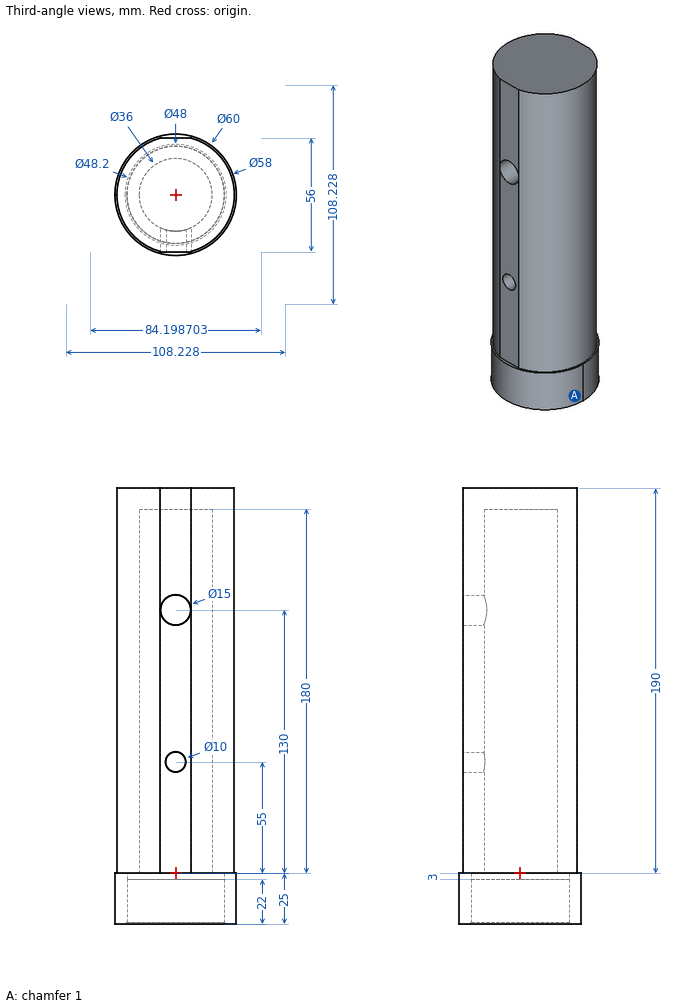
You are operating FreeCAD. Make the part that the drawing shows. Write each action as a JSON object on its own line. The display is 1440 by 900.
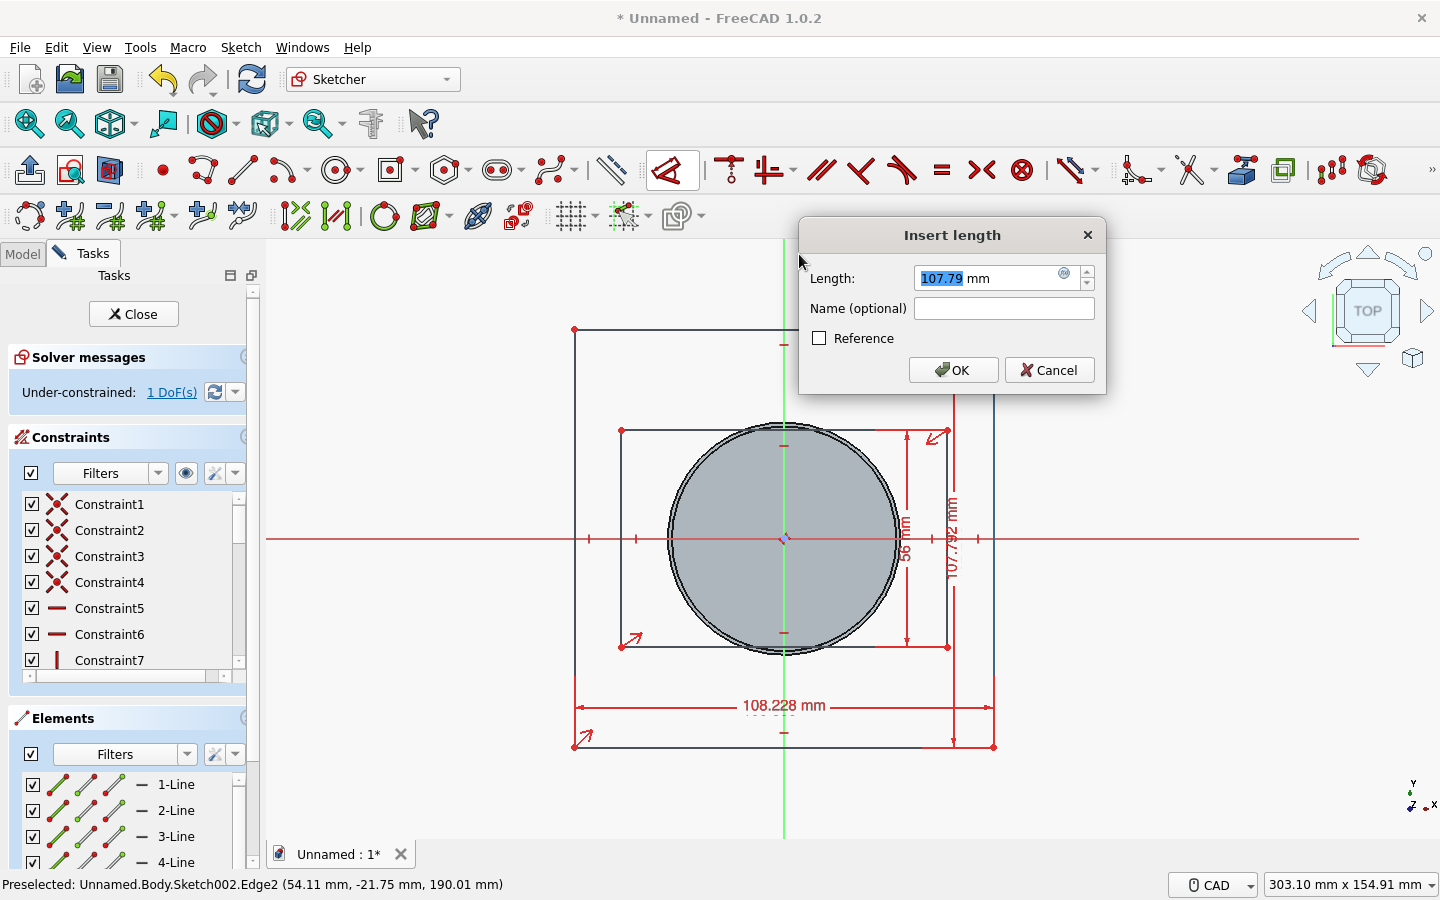
{"action": "type", "text": "108.228"}
{"action": "key", "text": "Return"}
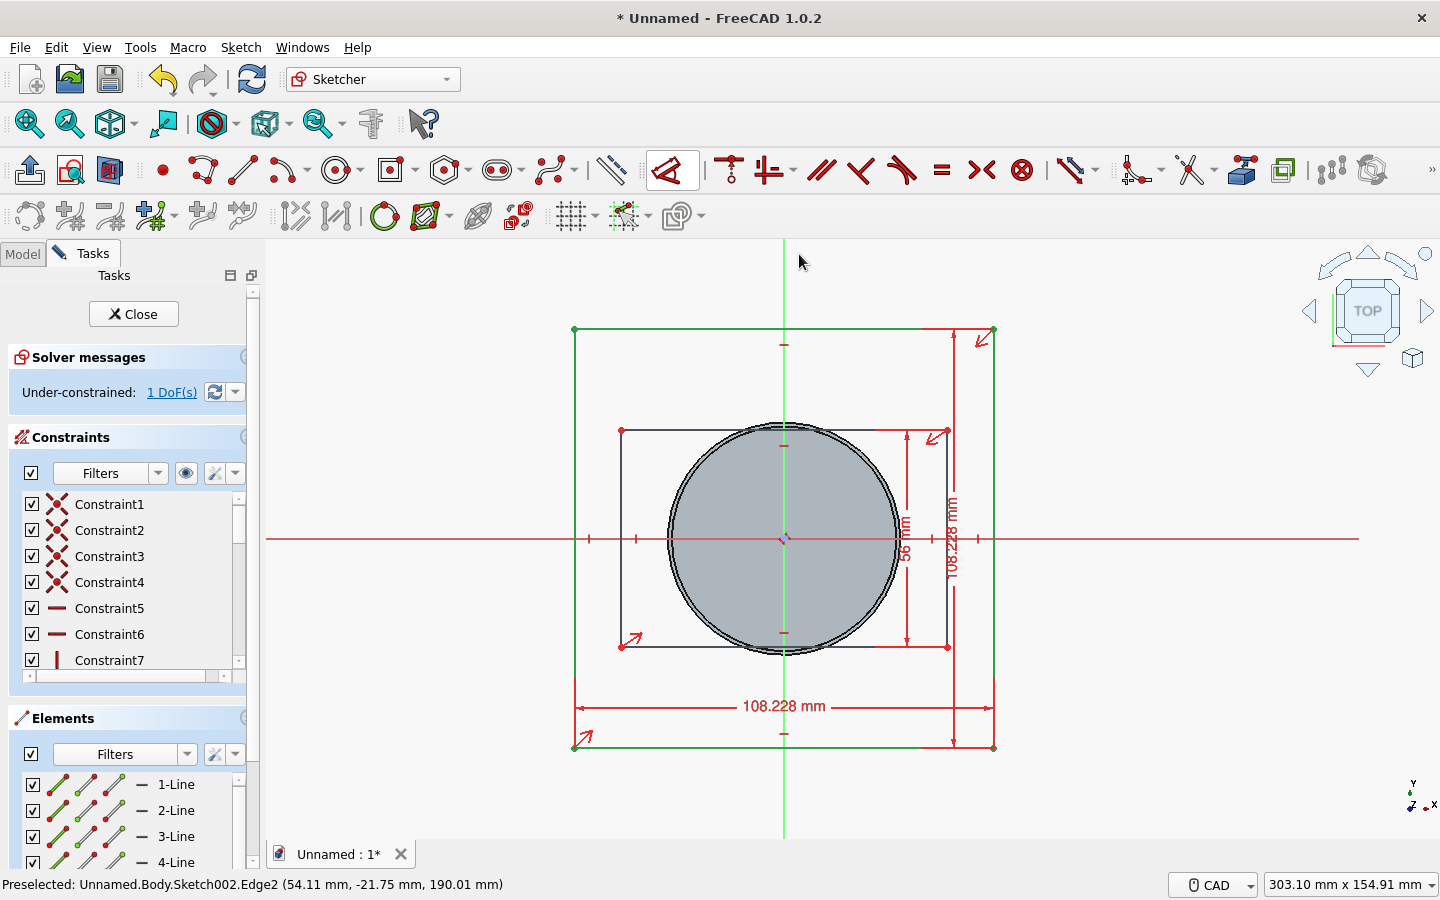
{"action": "left_click", "coordinate": [719, 647]}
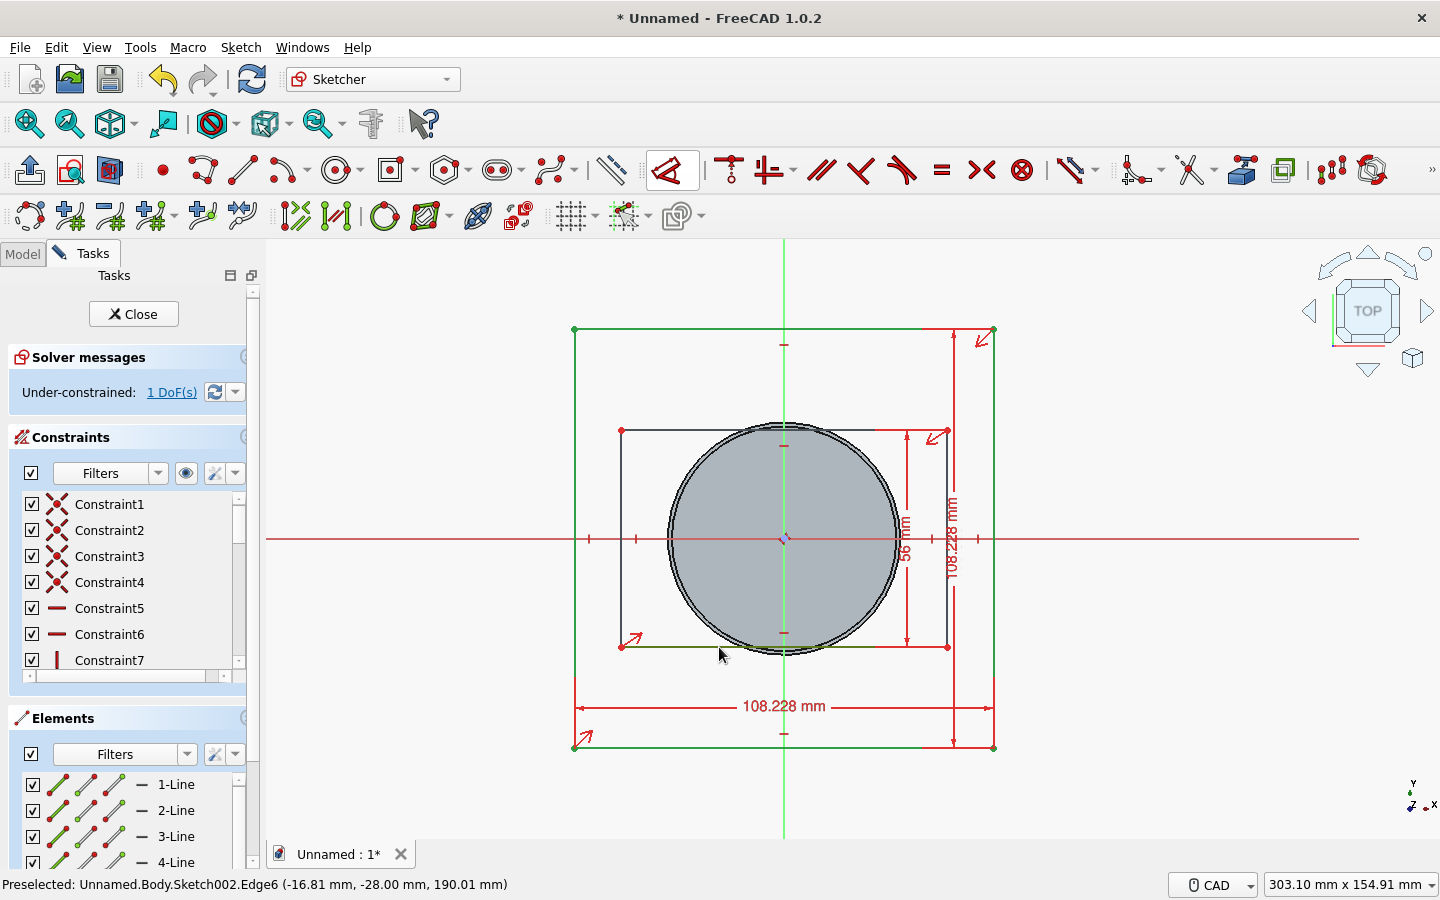
{"action": "key", "text": "l"}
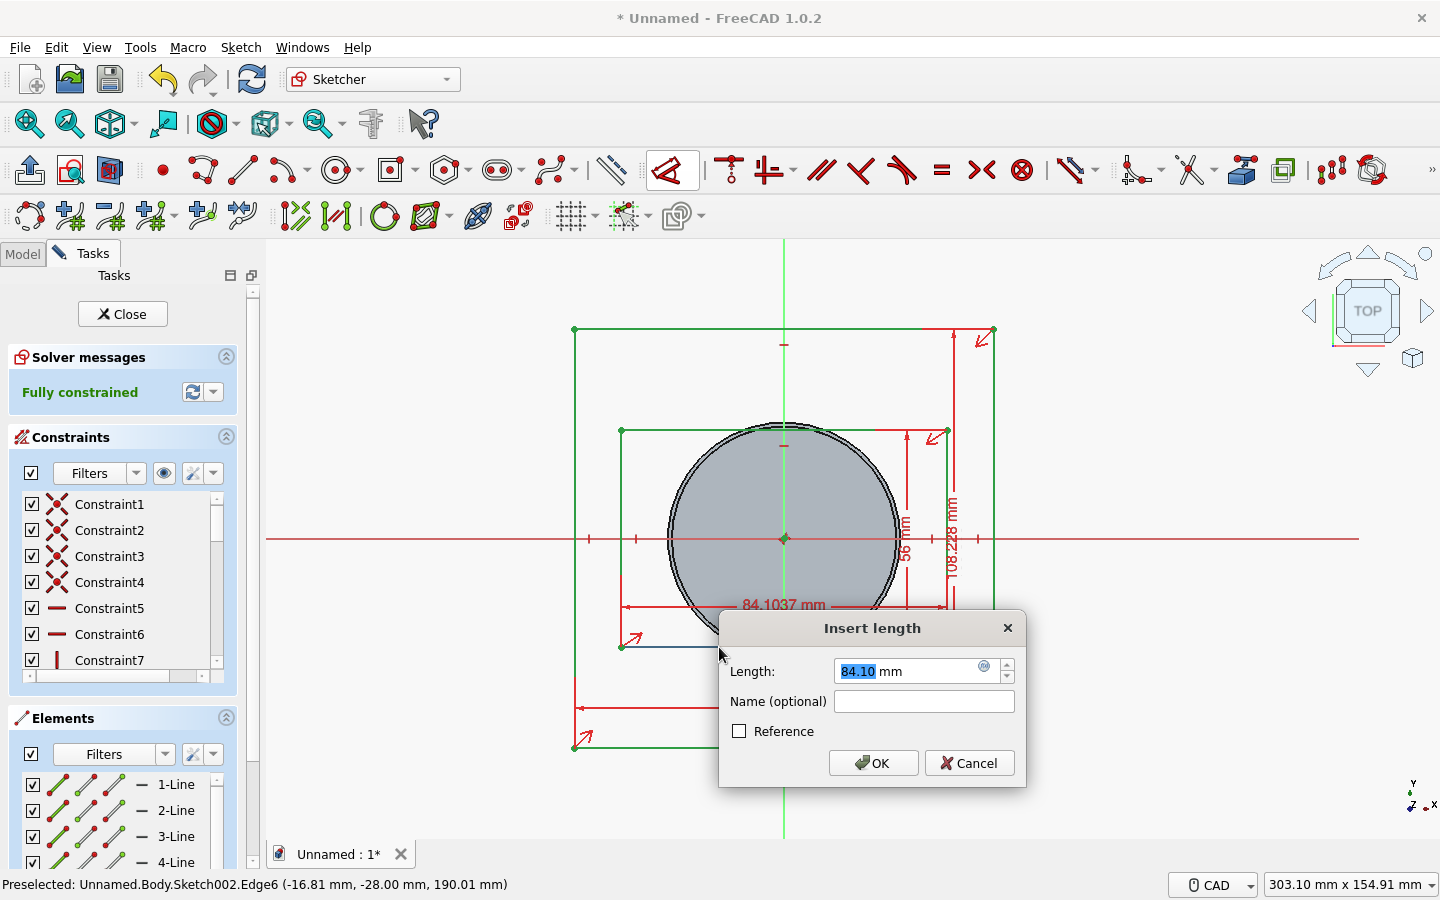
{"action": "type", "text": "84.198703"}
{"action": "key", "text": "Return"}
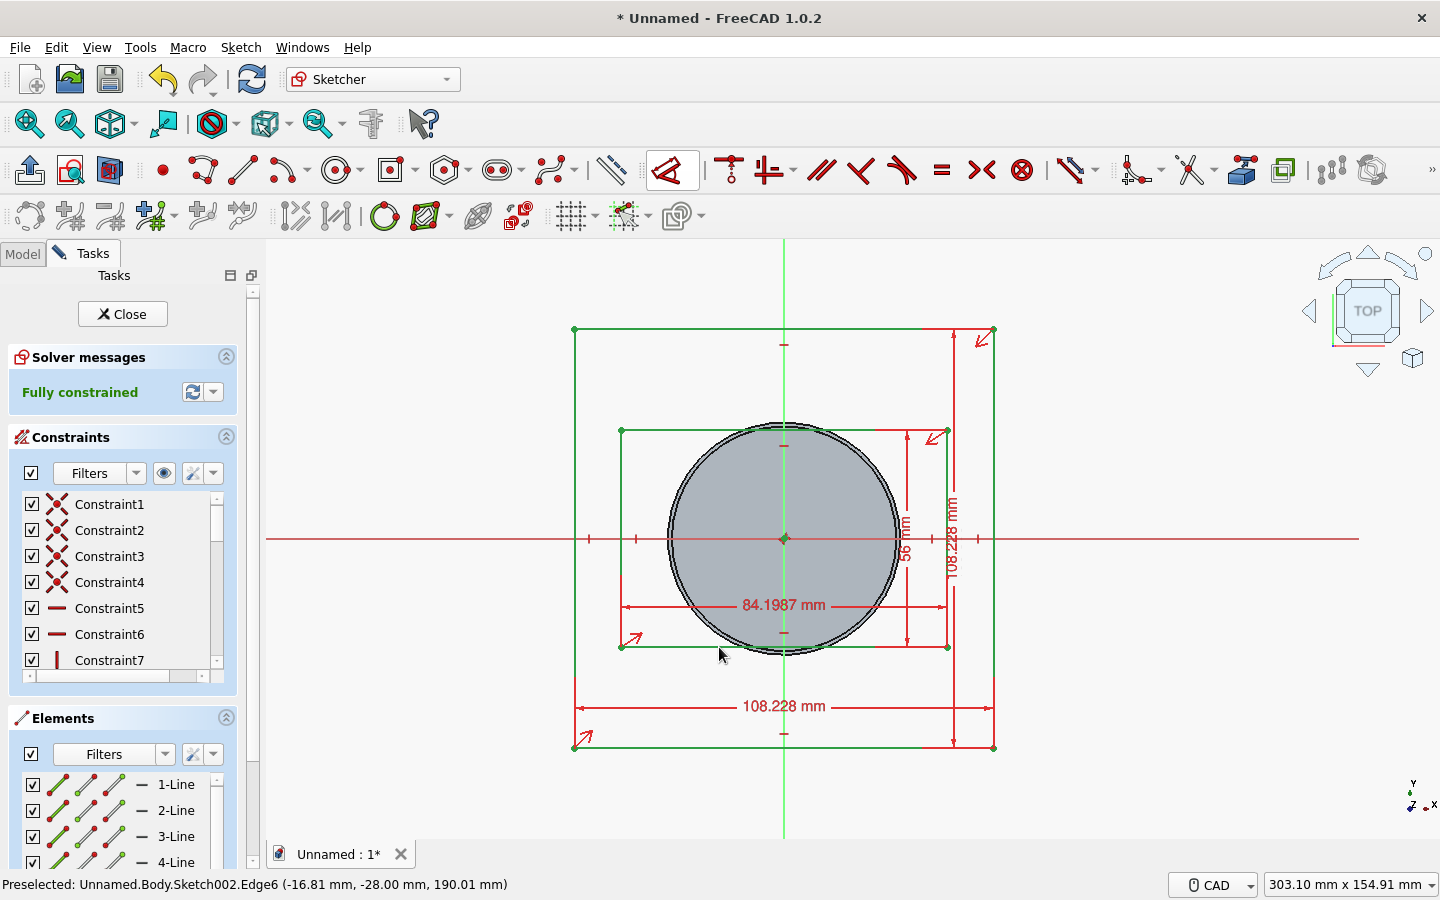
{"action": "left_click", "coordinate": [123, 314]}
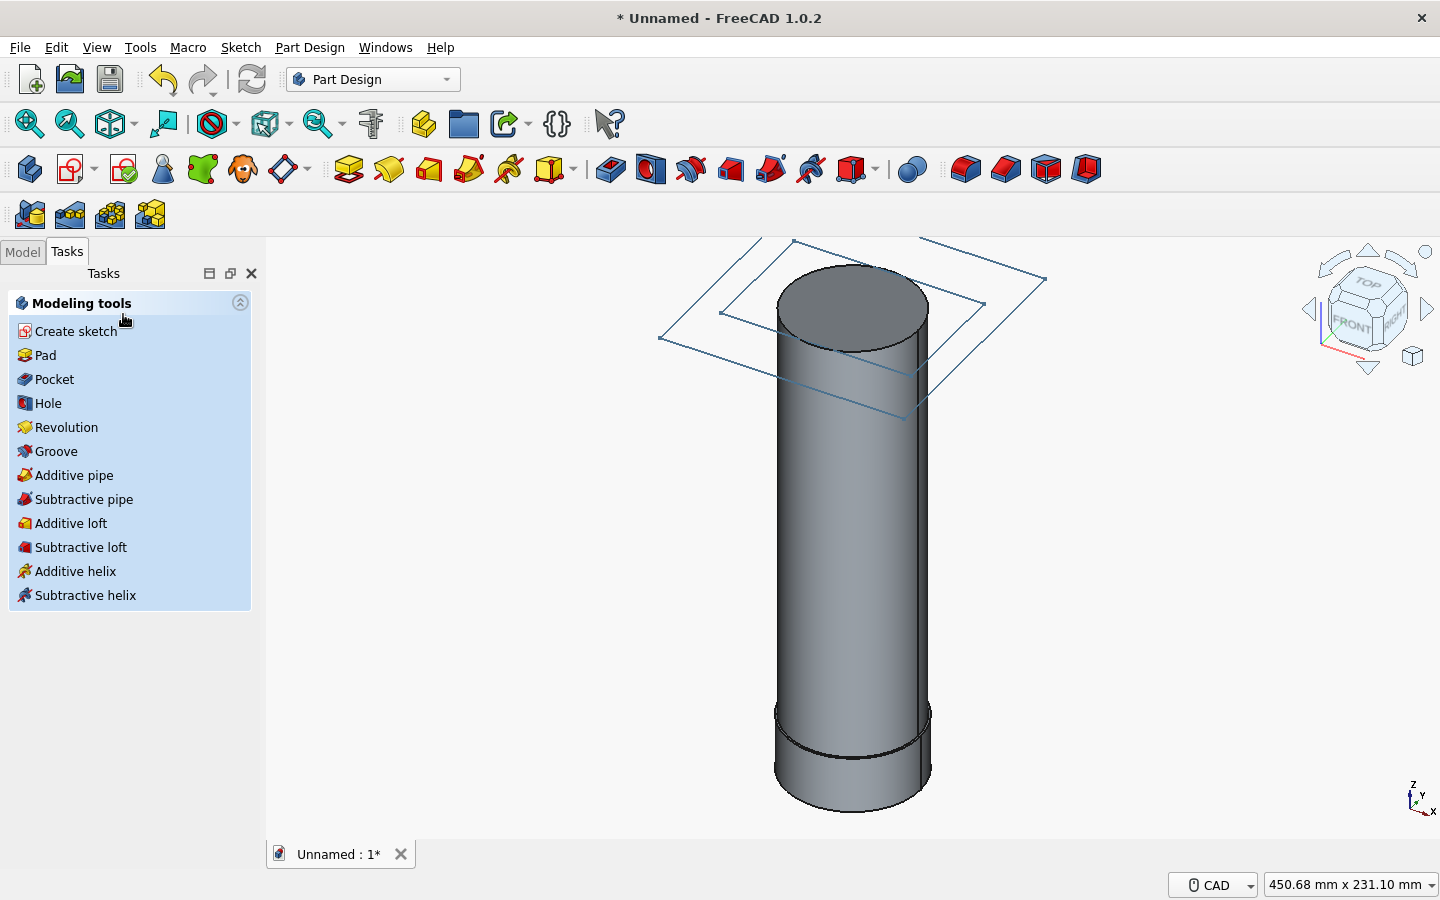
{"action": "left_click", "coordinate": [612, 170]}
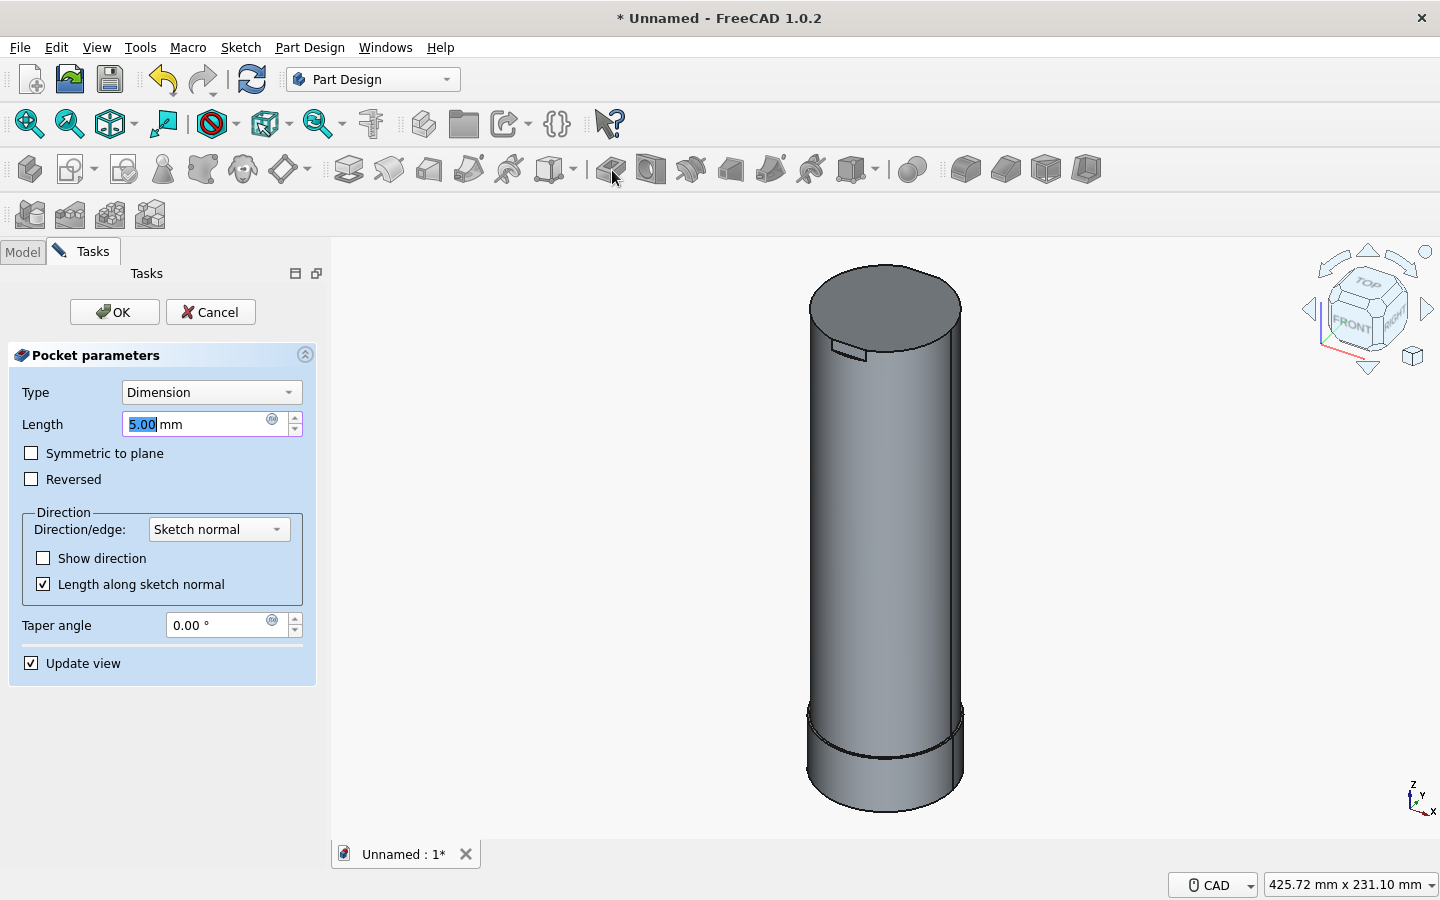
{"action": "type", "text": "190"}
{"action": "key", "text": "Tab"}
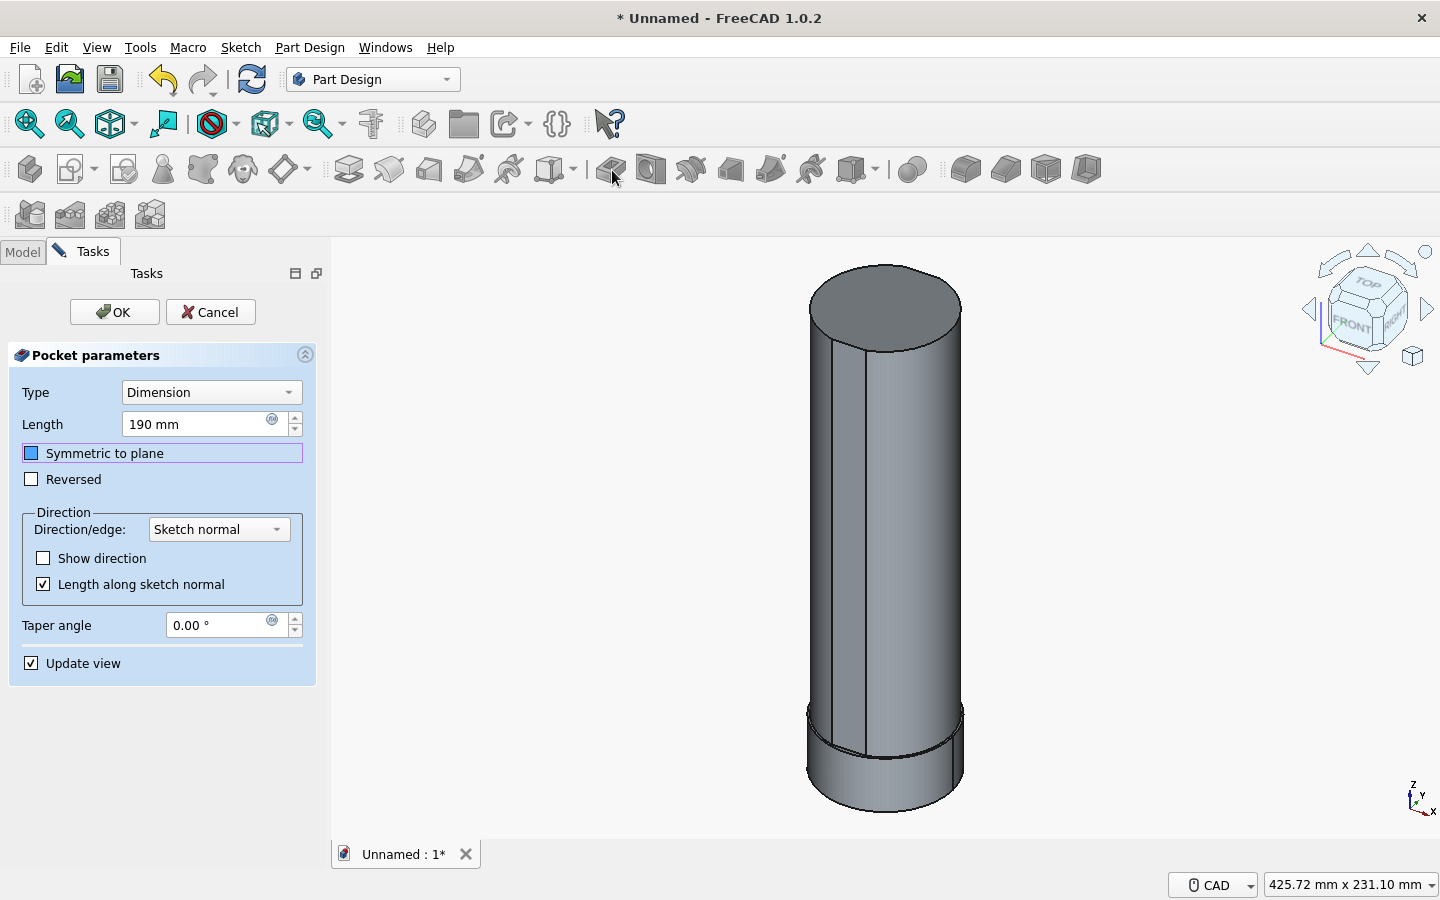
{"action": "left_click", "coordinate": [115, 312]}